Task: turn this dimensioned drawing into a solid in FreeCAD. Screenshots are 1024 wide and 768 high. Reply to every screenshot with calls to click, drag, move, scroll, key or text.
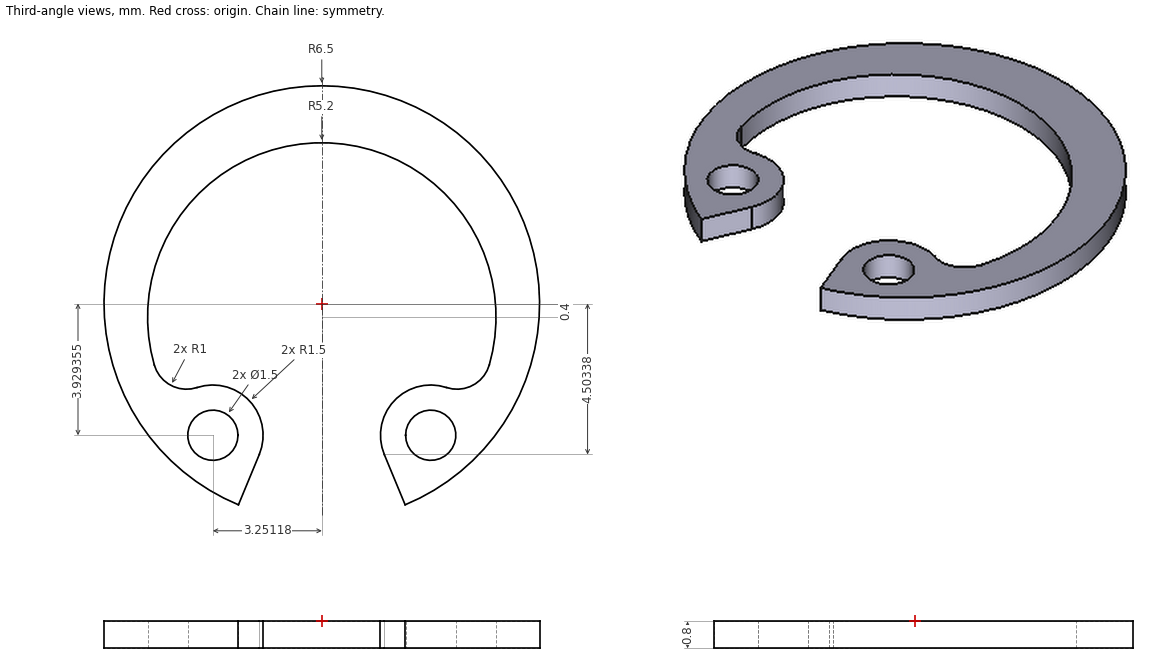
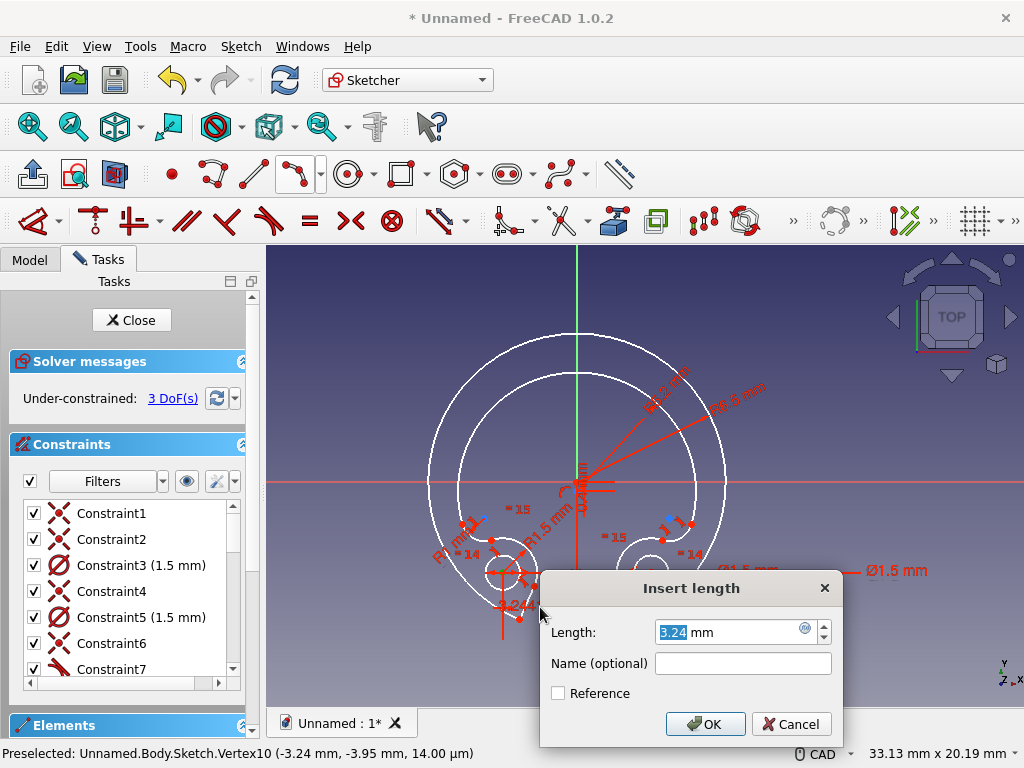
text(3.25118)
key(Return)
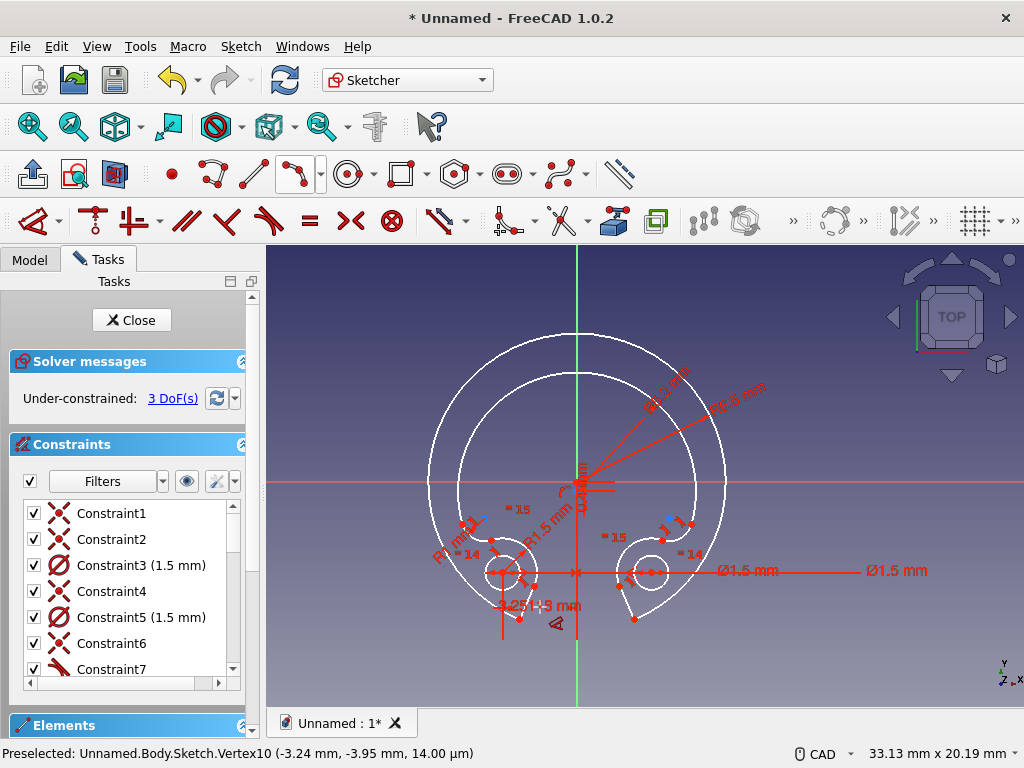
click(620, 586)
click(654, 510)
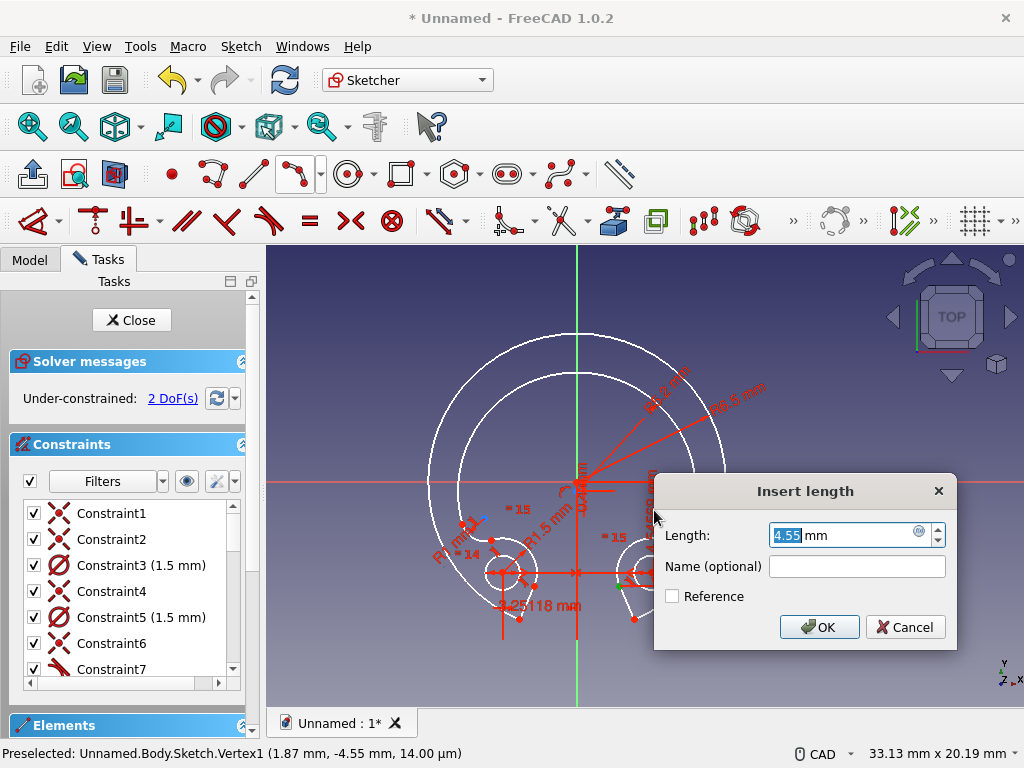
text(4.50338)
key(Return)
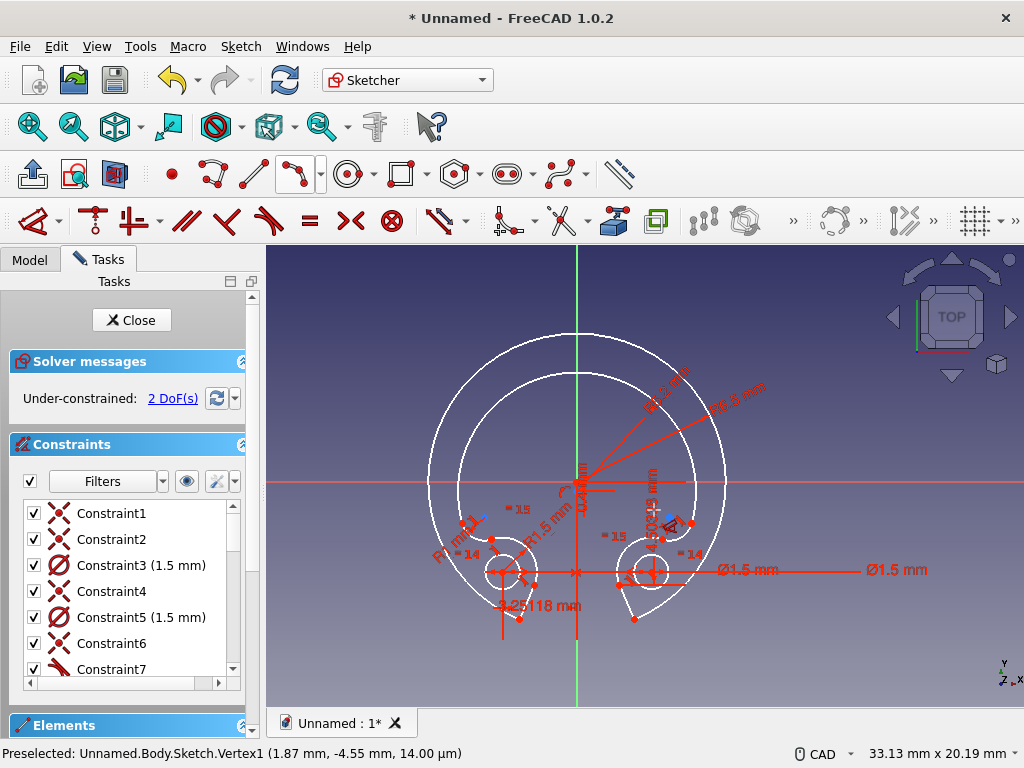
click(534, 585)
click(500, 498)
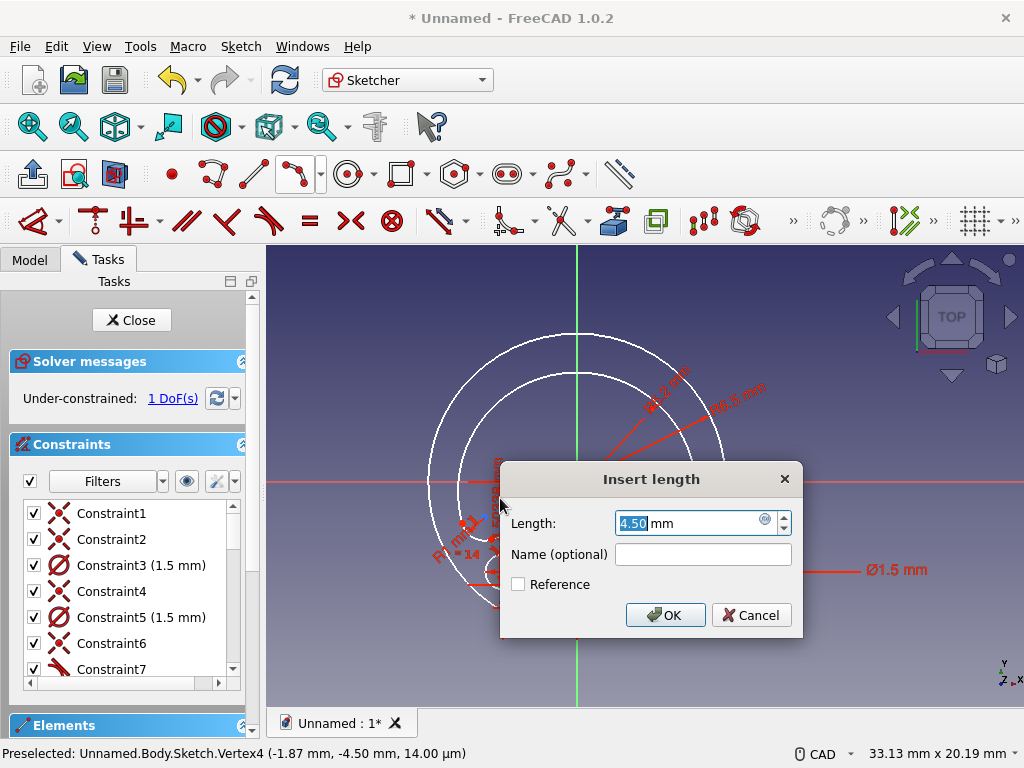
text(4.50338)
key(Return)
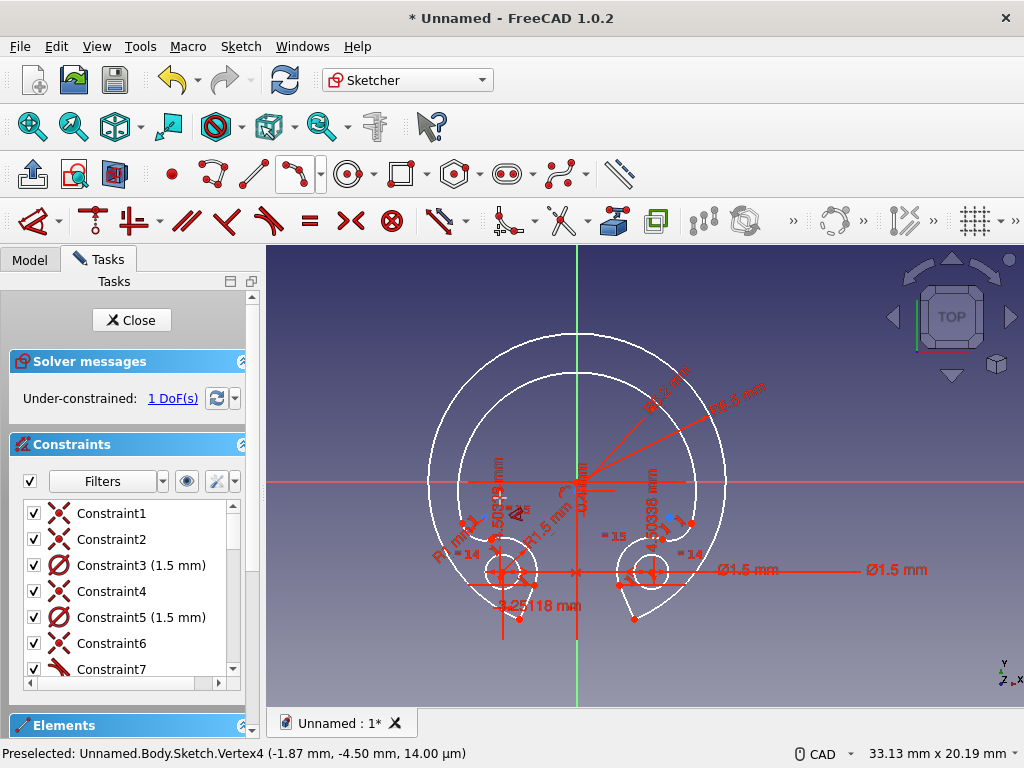
click(503, 572)
click(397, 507)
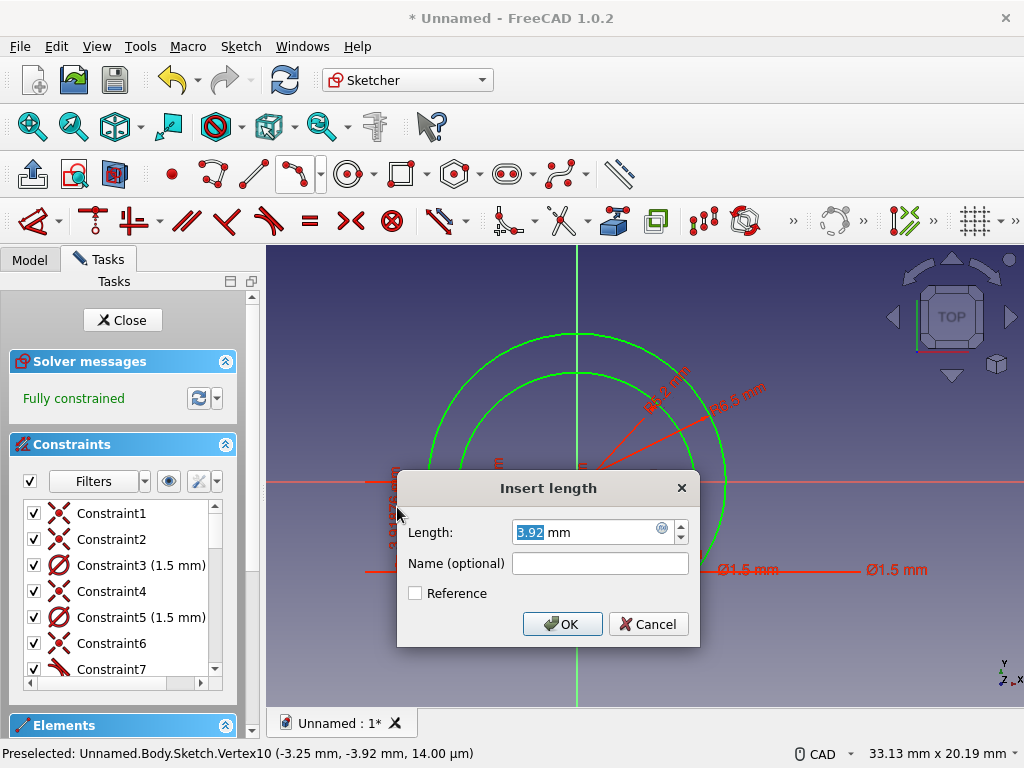
text(3.929355)
key(Return)
key(Escape)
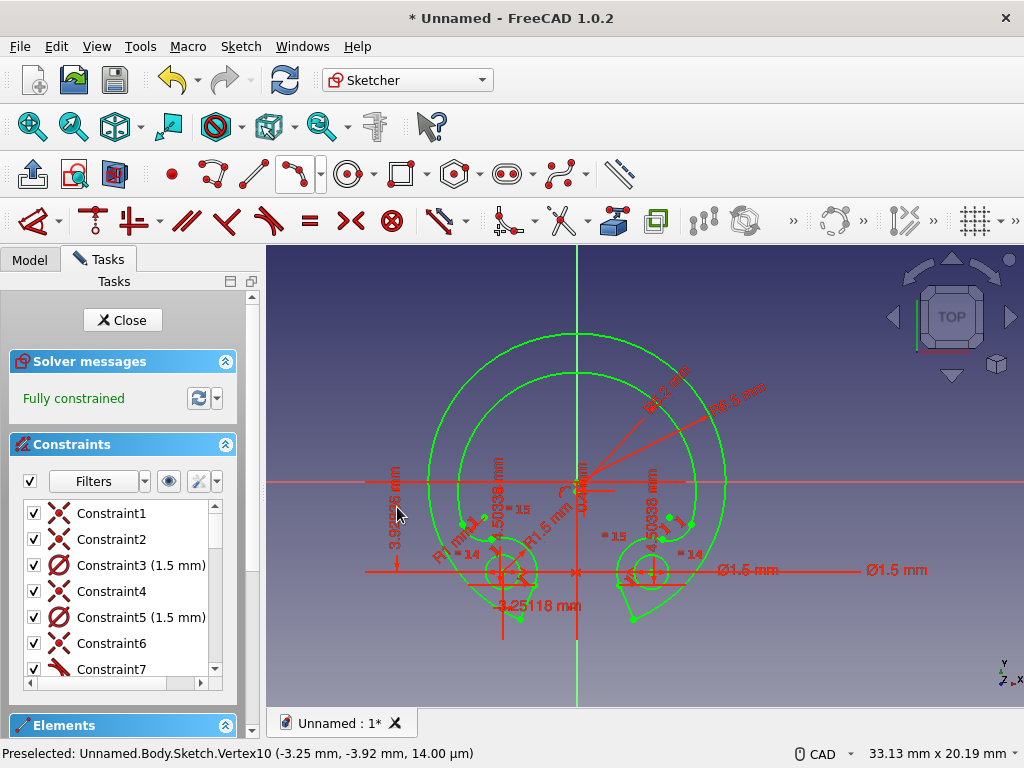
click(123, 320)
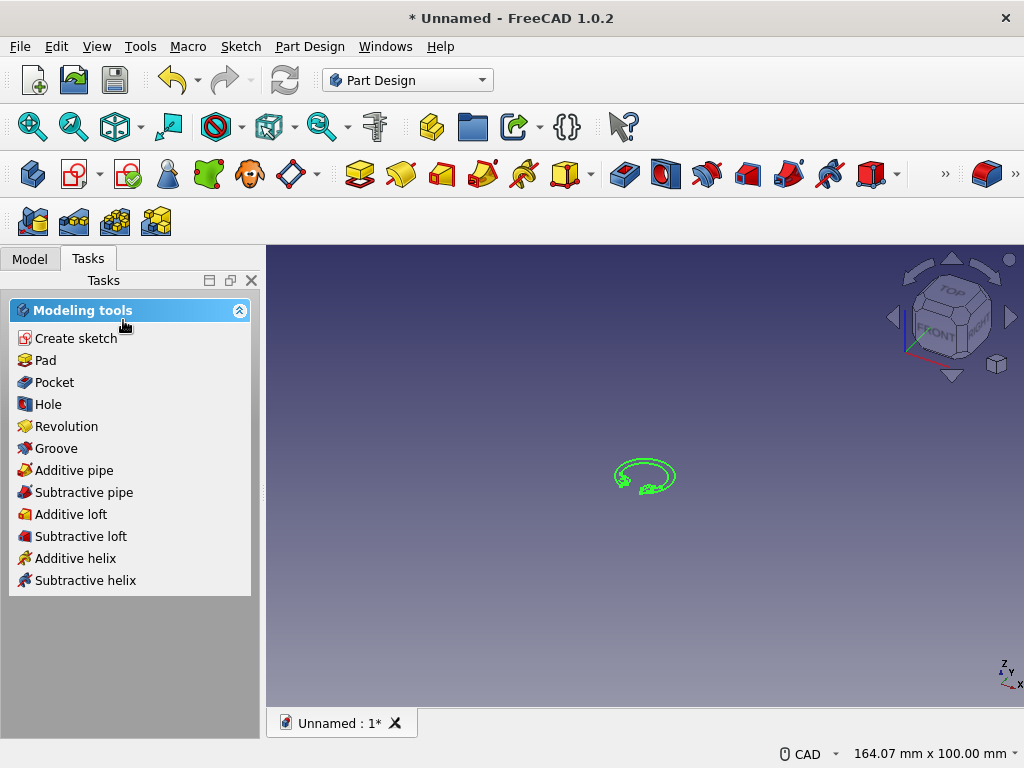
click(360, 174)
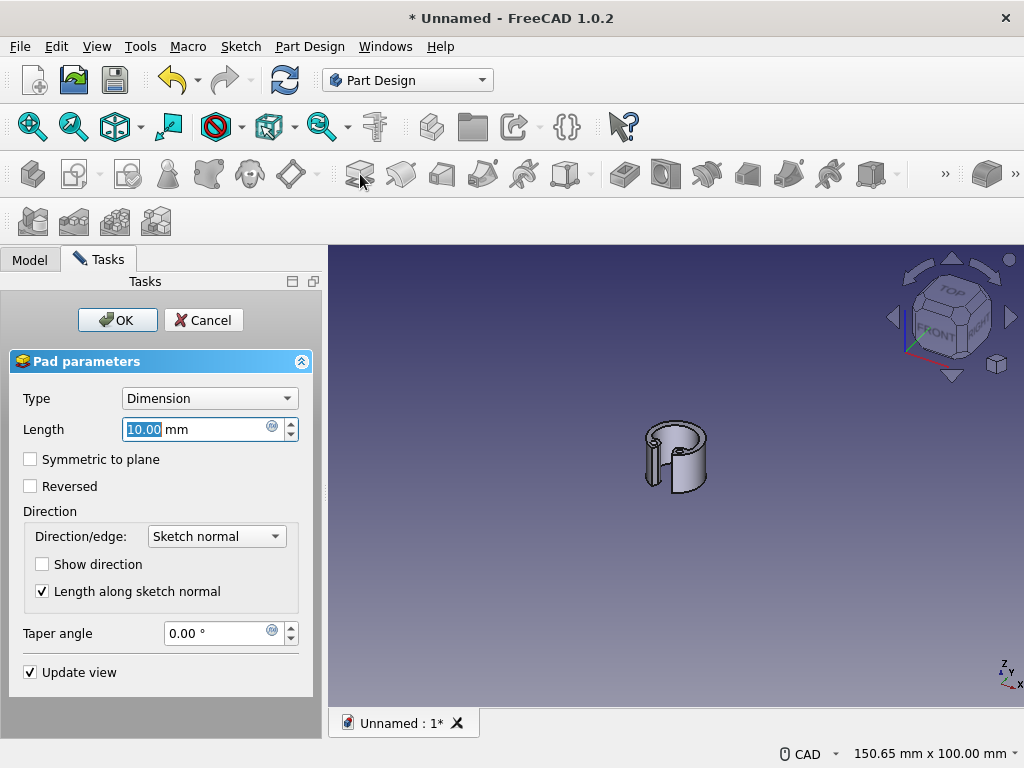
text(0.8)
key(Tab)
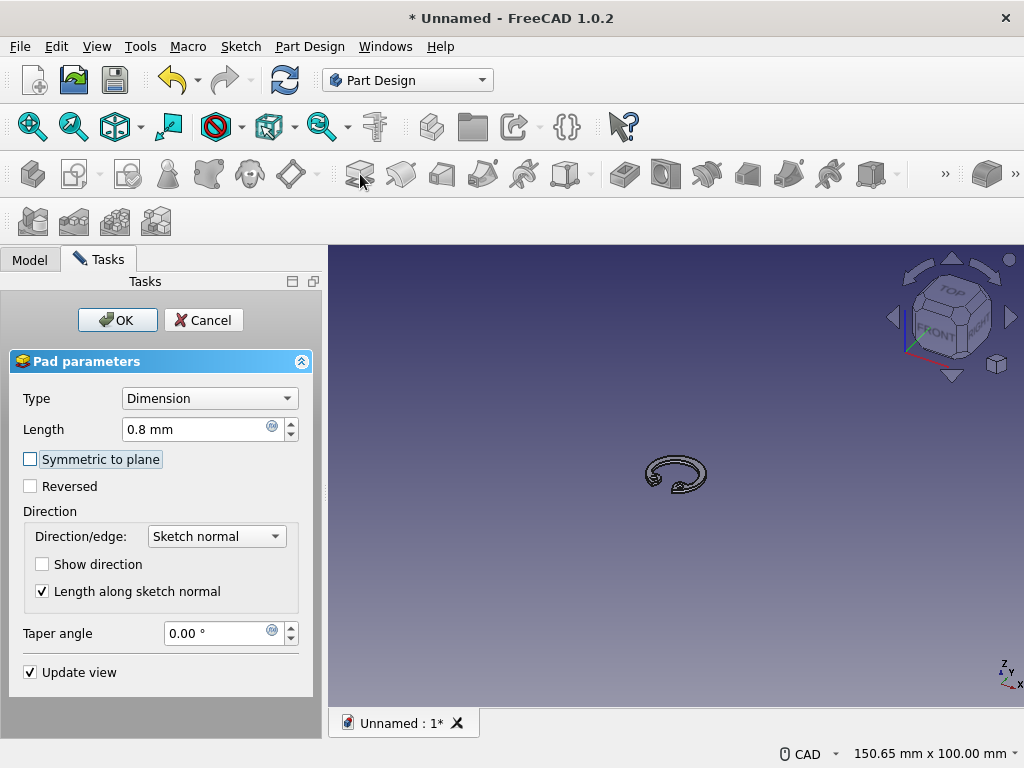
click(31, 486)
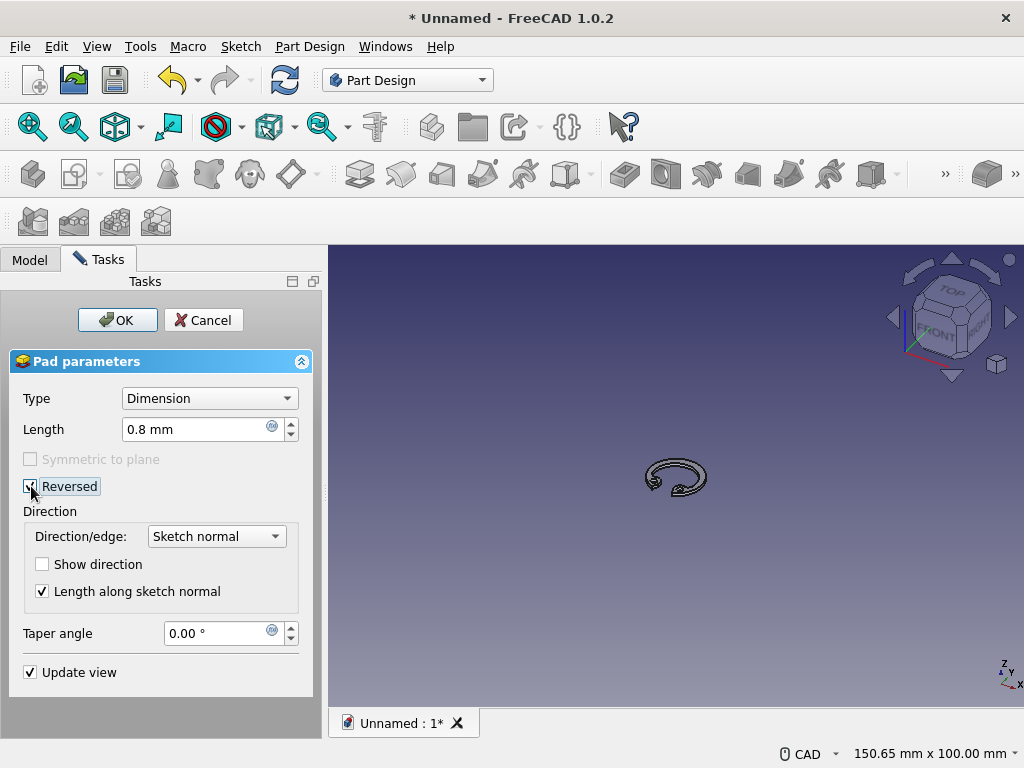
click(118, 320)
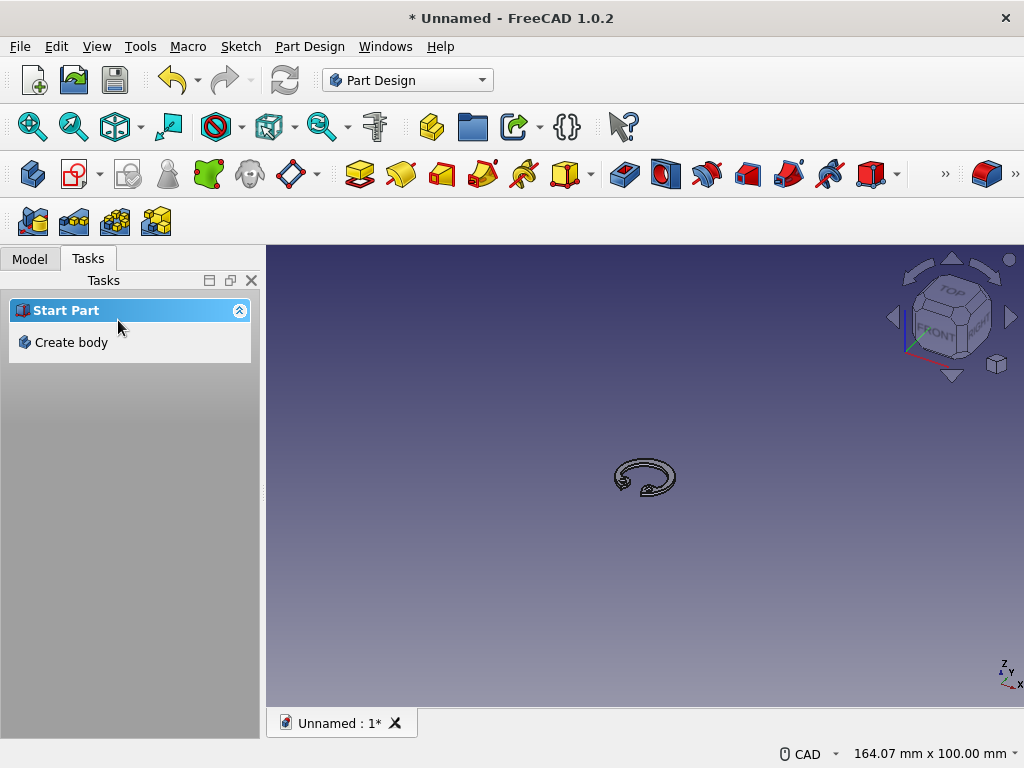
key(0)